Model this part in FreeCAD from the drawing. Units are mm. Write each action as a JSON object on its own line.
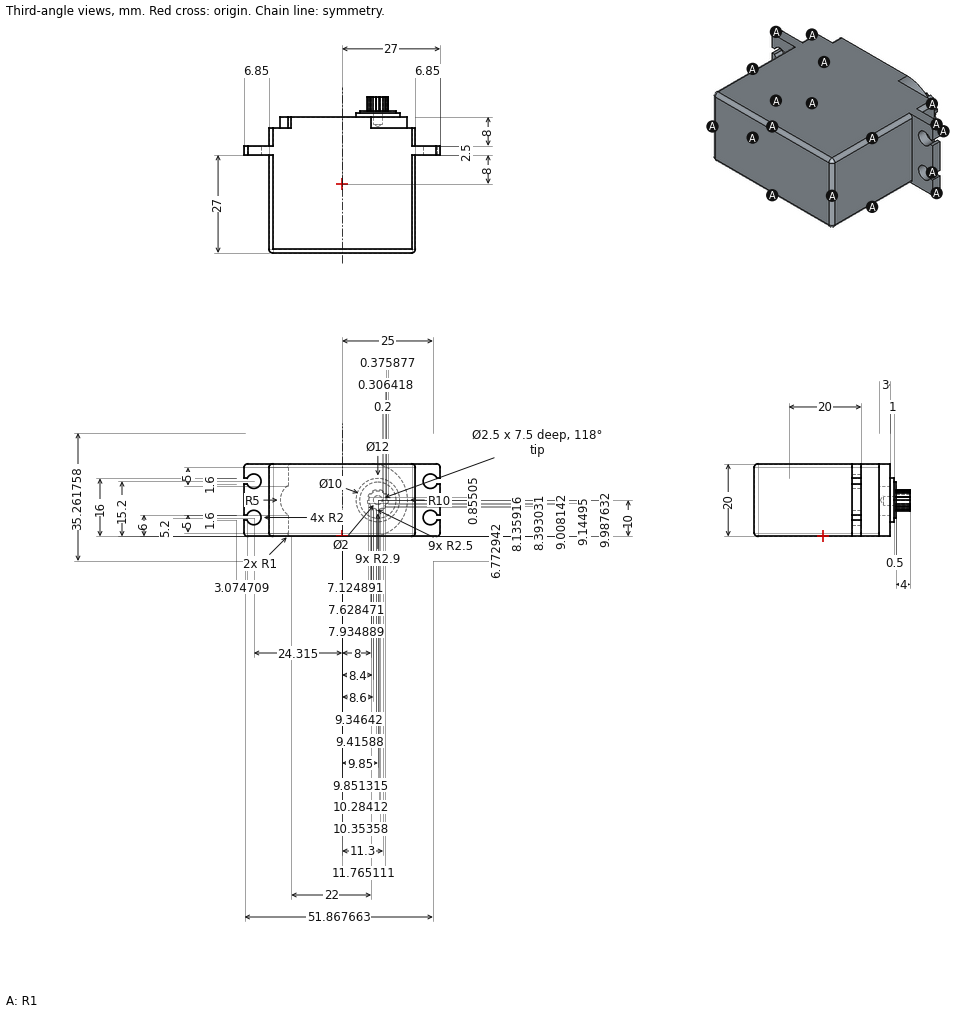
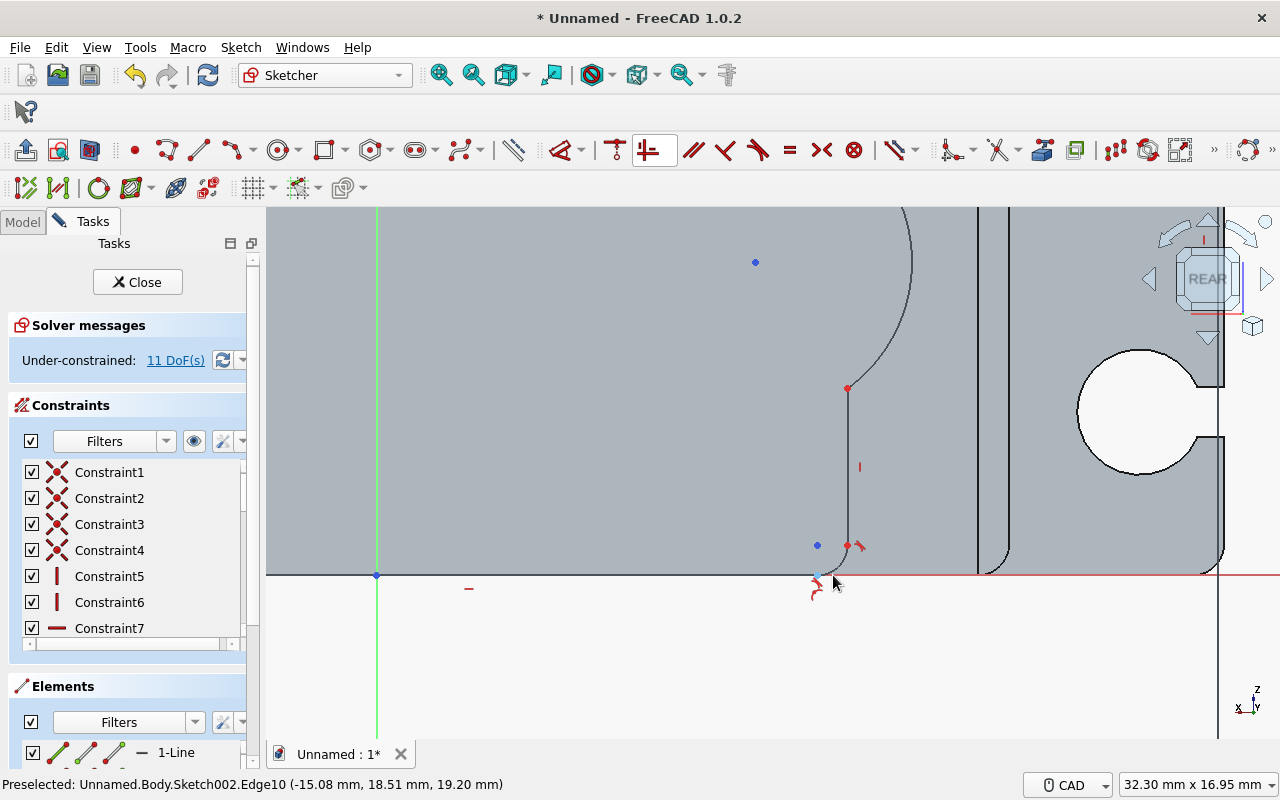
{"action": "left_click", "coordinate": [831, 572]}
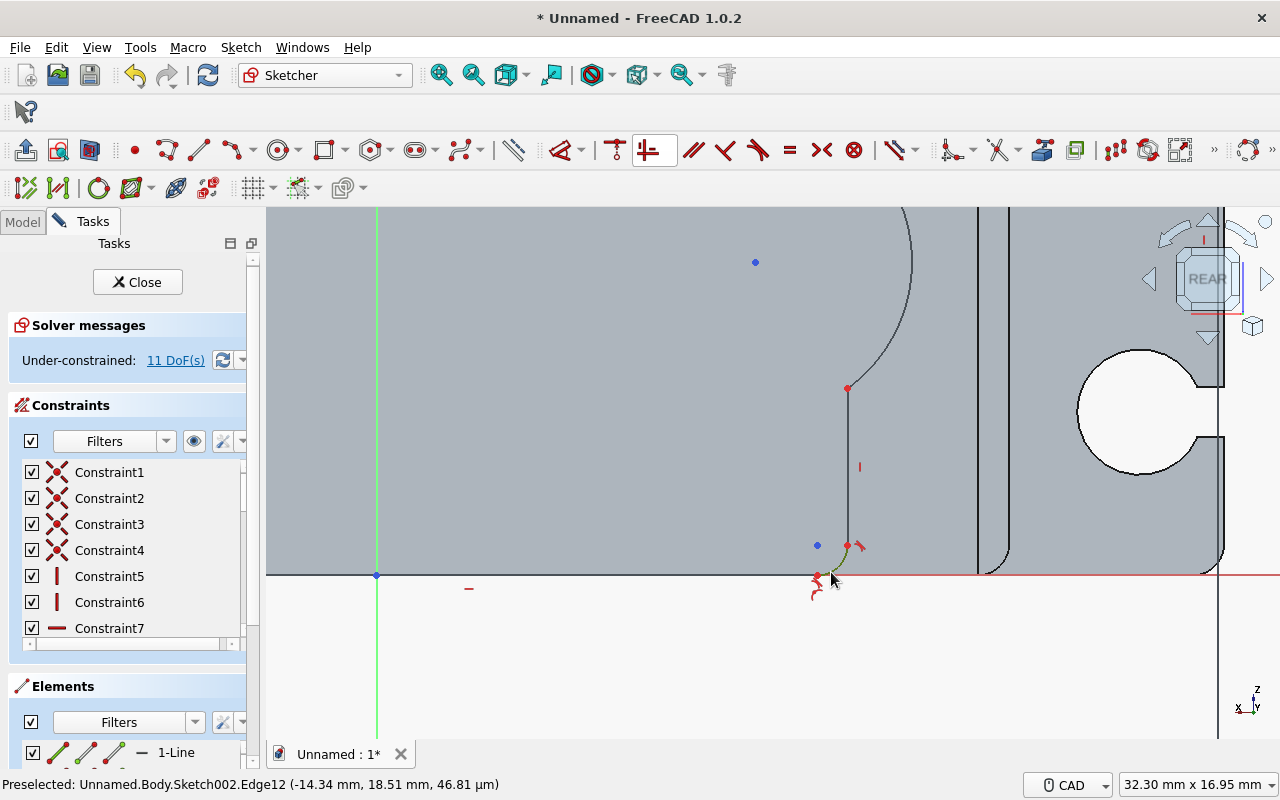
{"action": "left_click", "coordinate": [790, 150]}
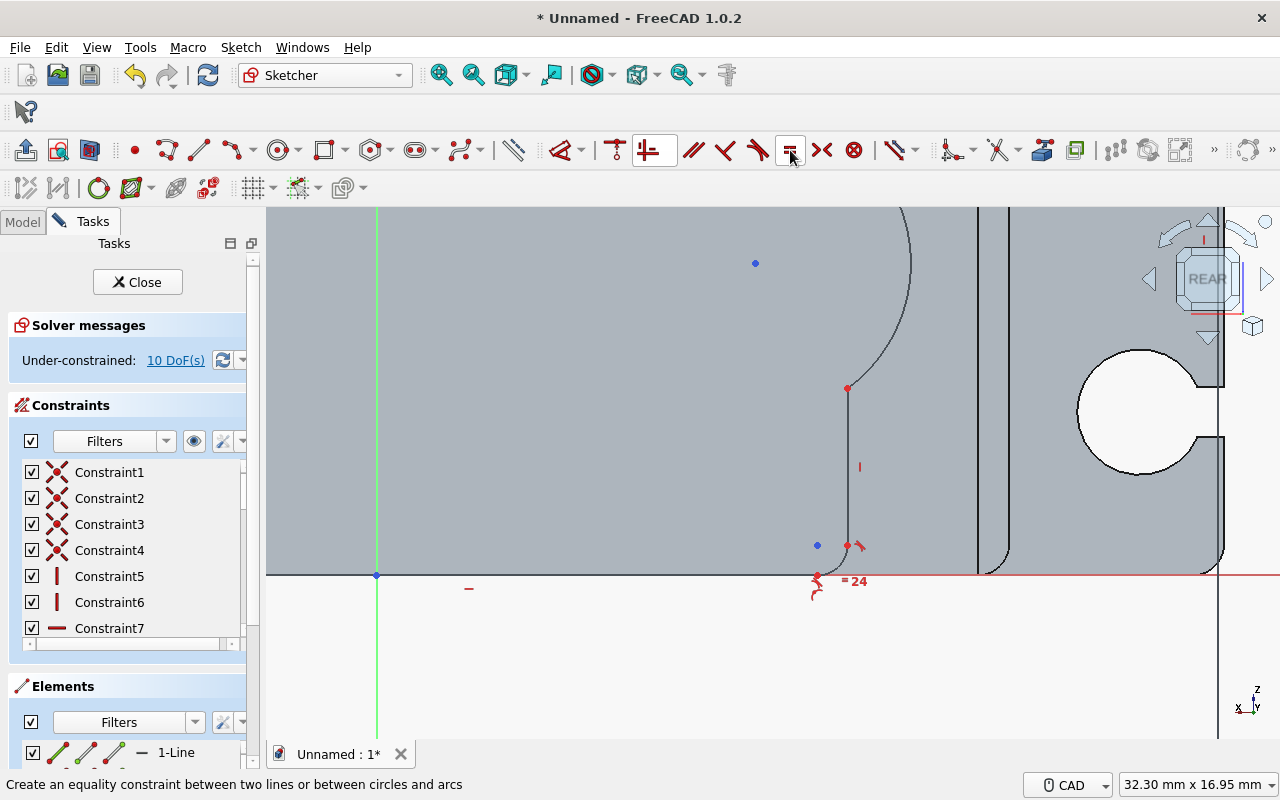
{"action": "left_click", "coordinate": [560, 150]}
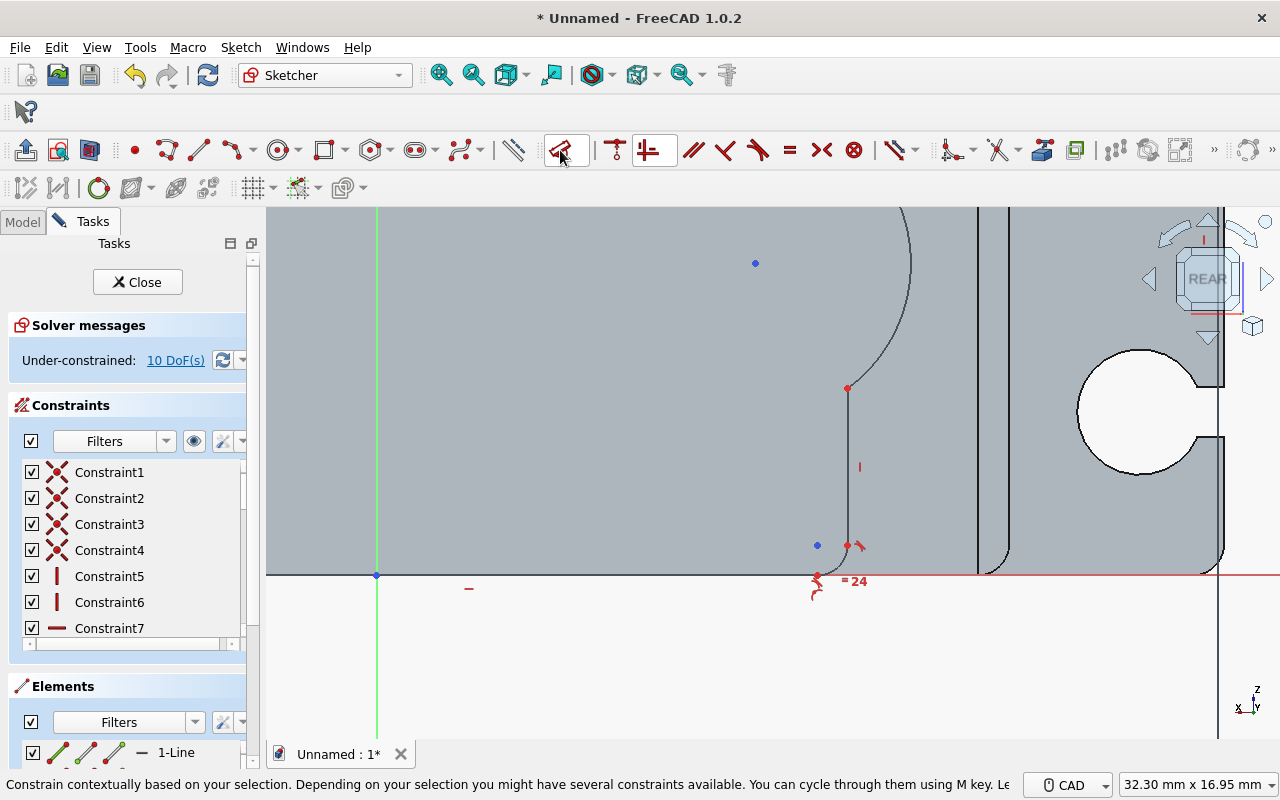
{"action": "scroll", "coordinate": [833, 576], "scroll_direction": "down", "scroll_amount": 6}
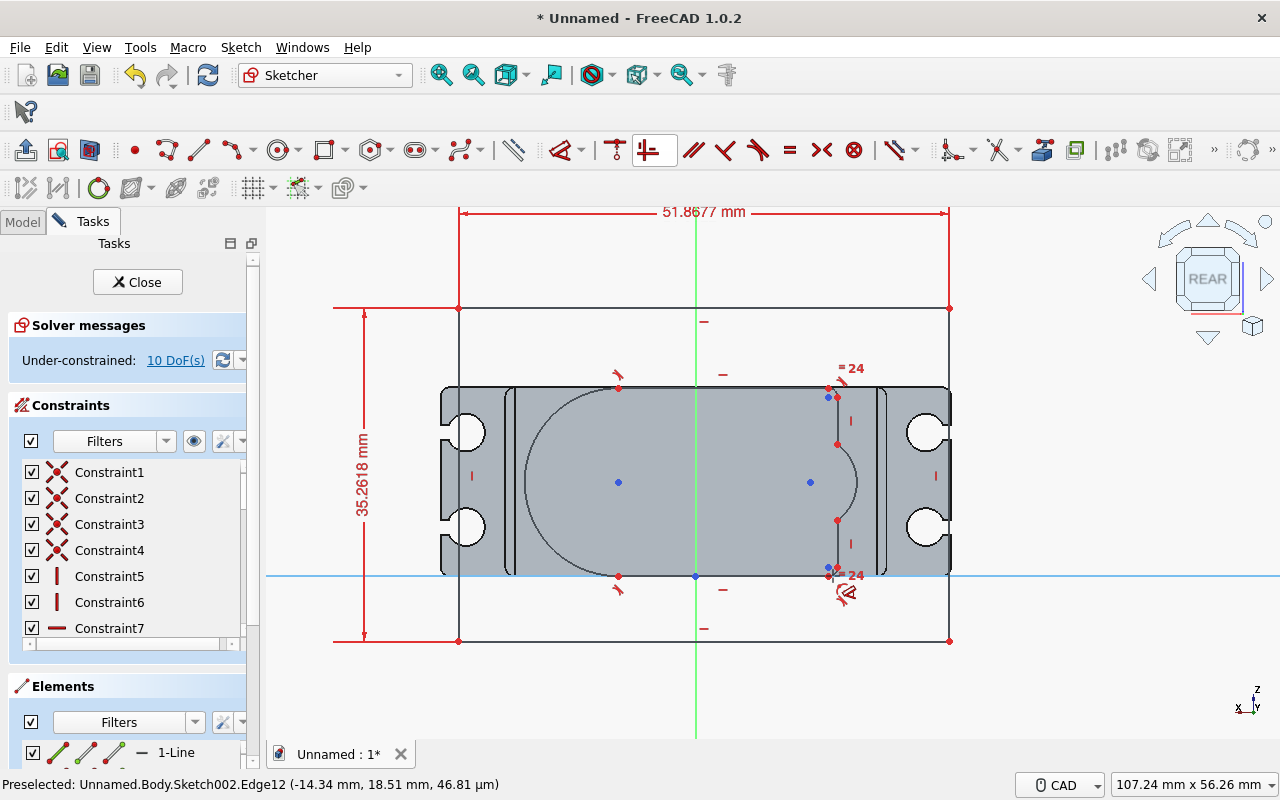
{"action": "left_click", "coordinate": [543, 427]}
{"action": "left_click", "coordinate": [517, 408]}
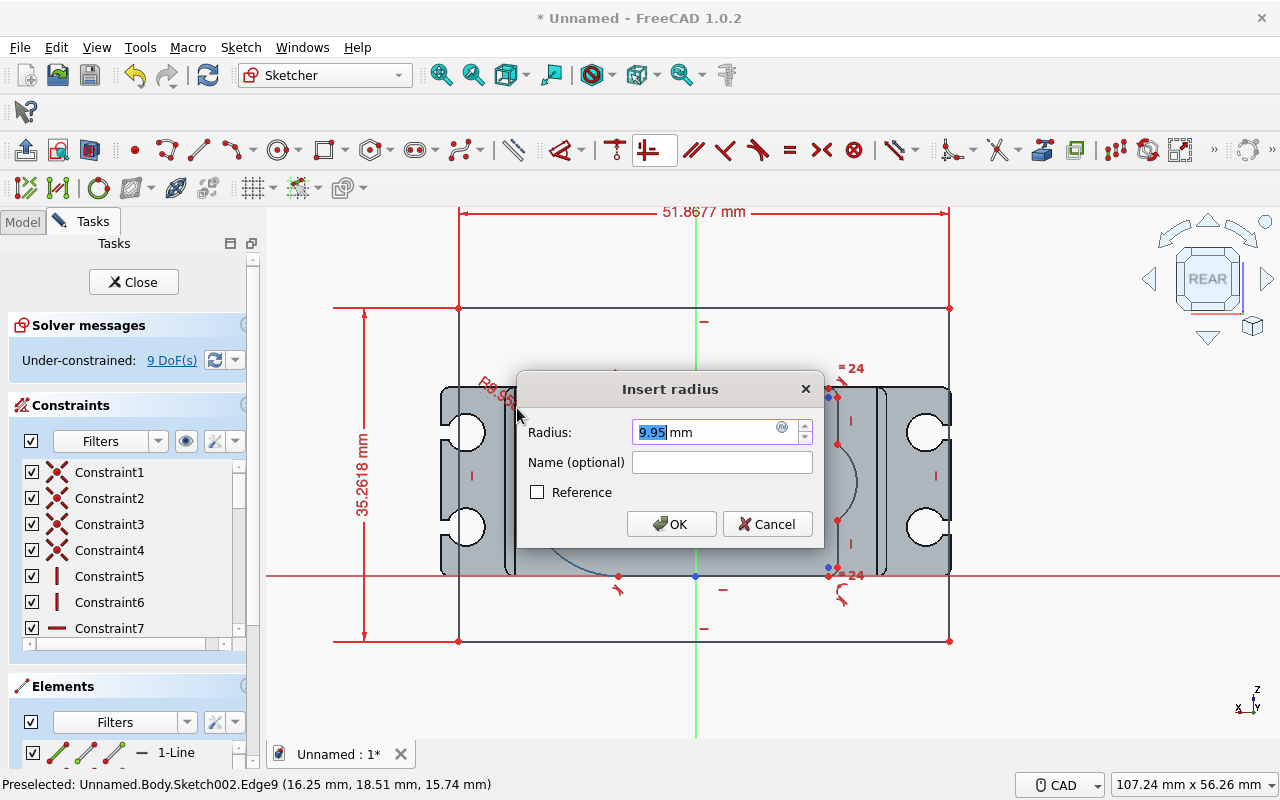
{"action": "type", "text": "10"}
{"action": "key", "text": "Return"}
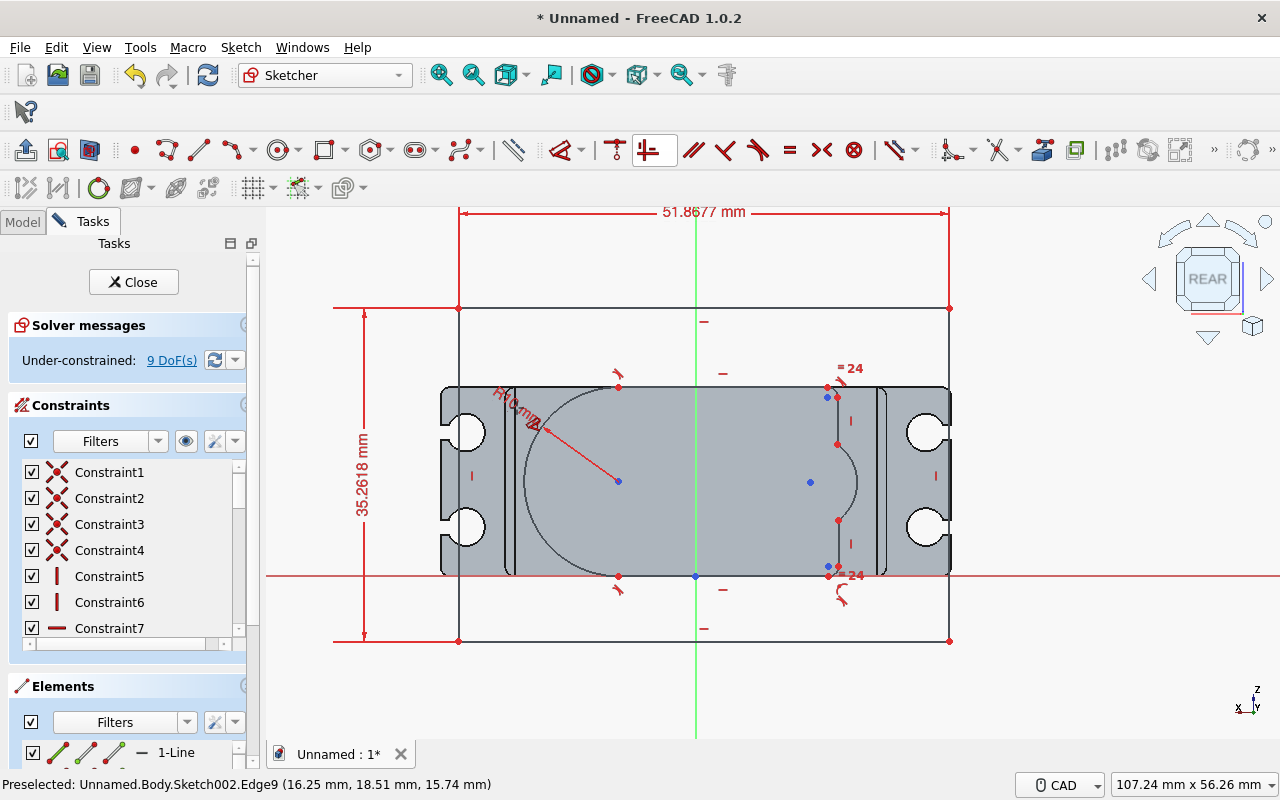
{"action": "scroll", "coordinate": [835, 390], "scroll_direction": "up", "scroll_amount": 8}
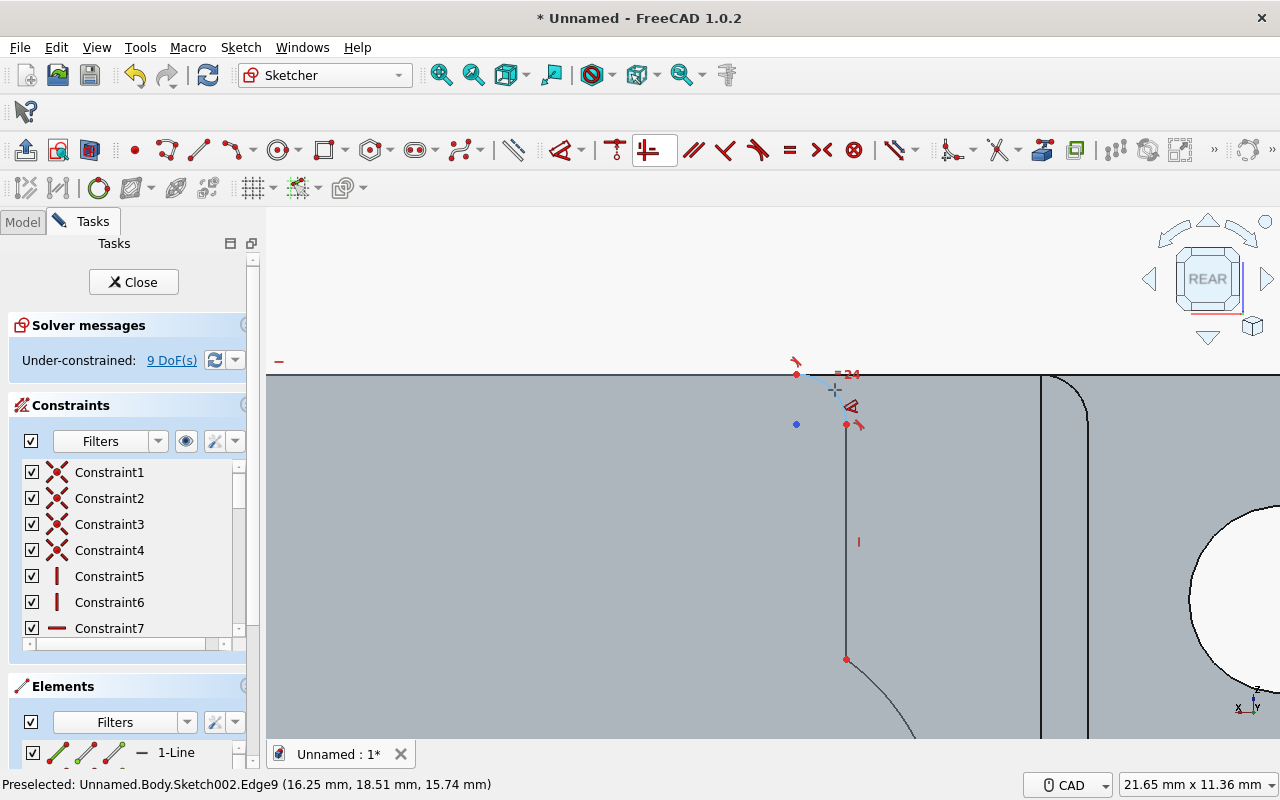
{"action": "left_click", "coordinate": [832, 389]}
{"action": "left_click", "coordinate": [855, 366]}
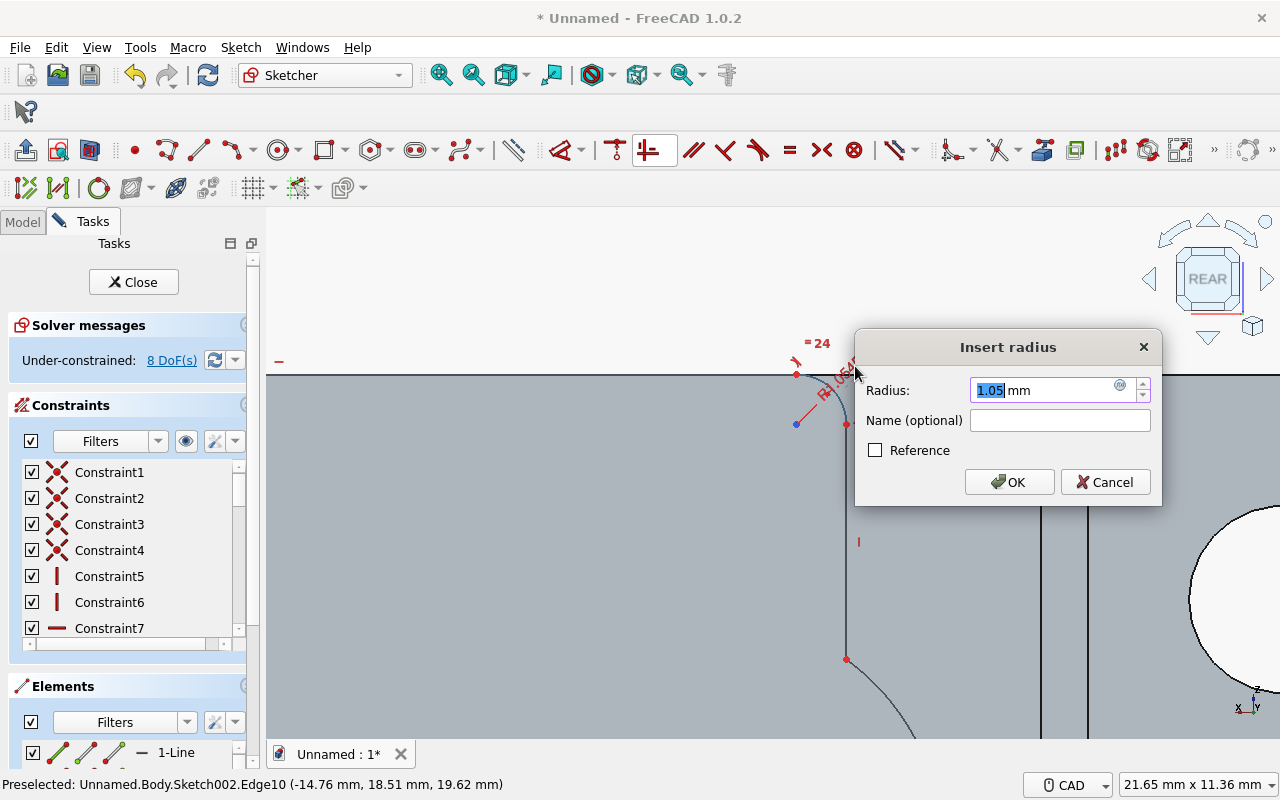
{"action": "type", "text": "1"}
{"action": "key", "text": "Return"}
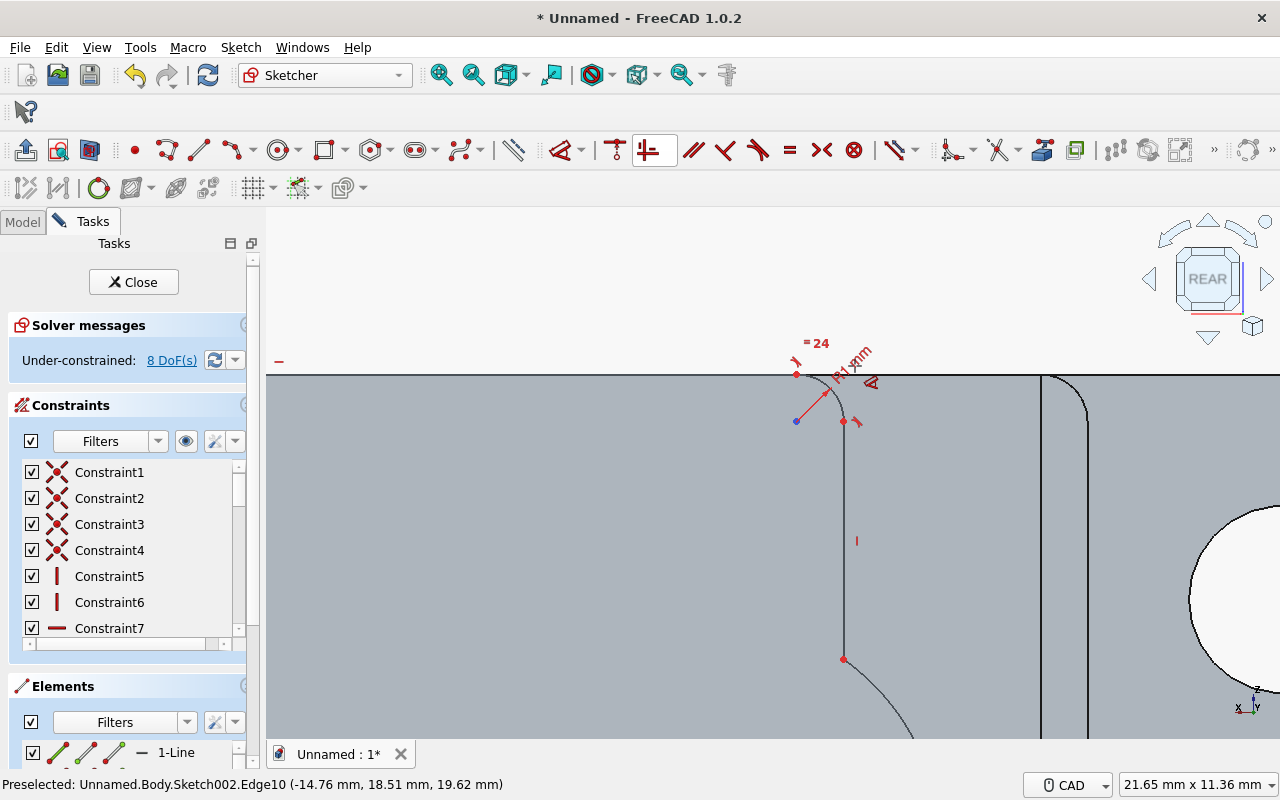
{"action": "scroll", "coordinate": [835, 390], "scroll_direction": "down", "scroll_amount": 8}